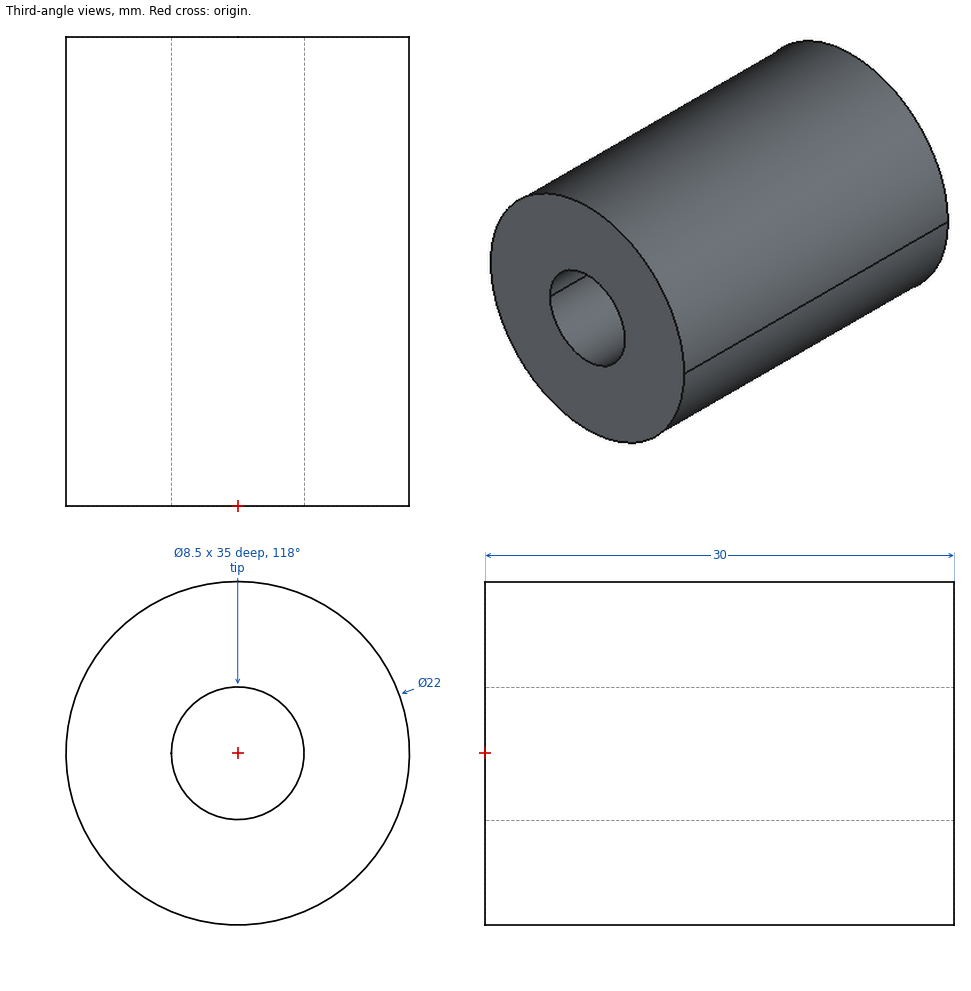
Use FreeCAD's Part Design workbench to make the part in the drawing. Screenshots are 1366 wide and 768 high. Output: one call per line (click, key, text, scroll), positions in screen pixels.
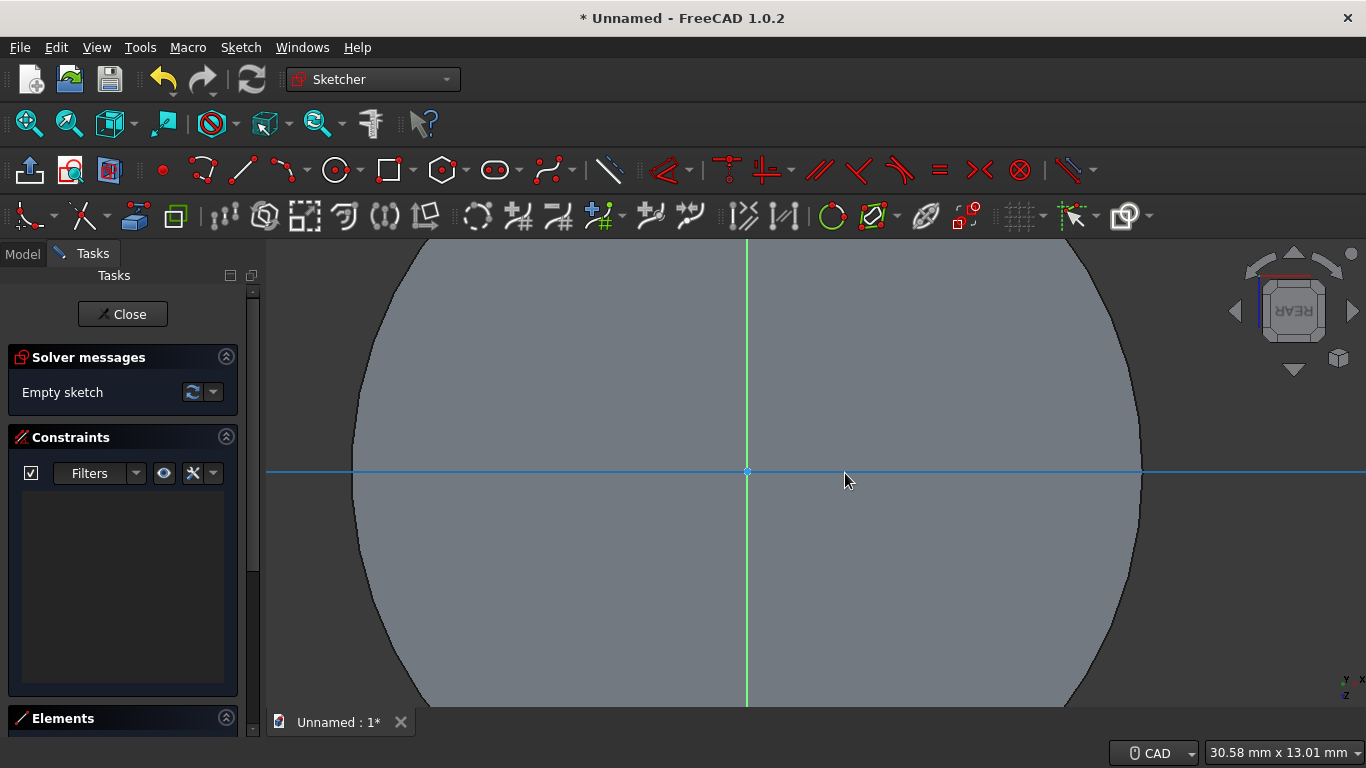
click(336, 170)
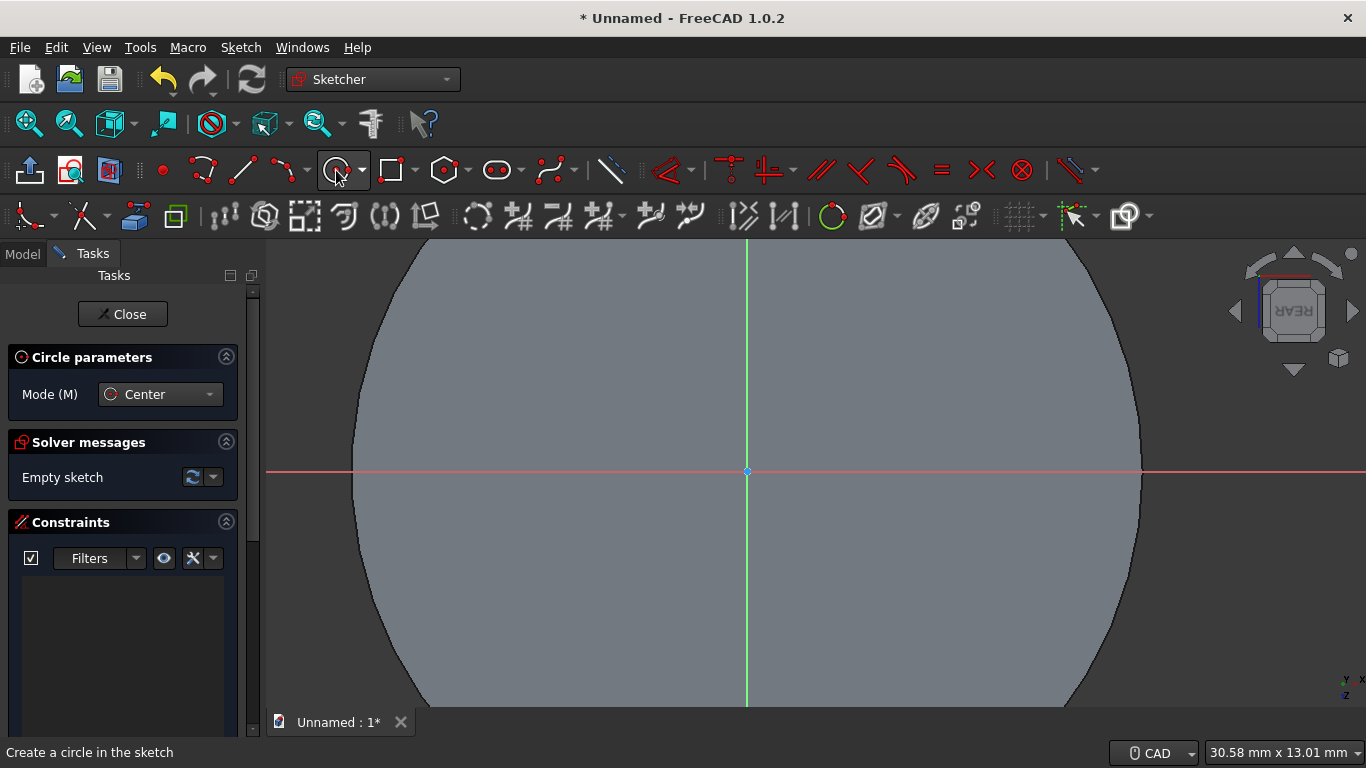
click(747, 472)
click(855, 364)
key(Escape)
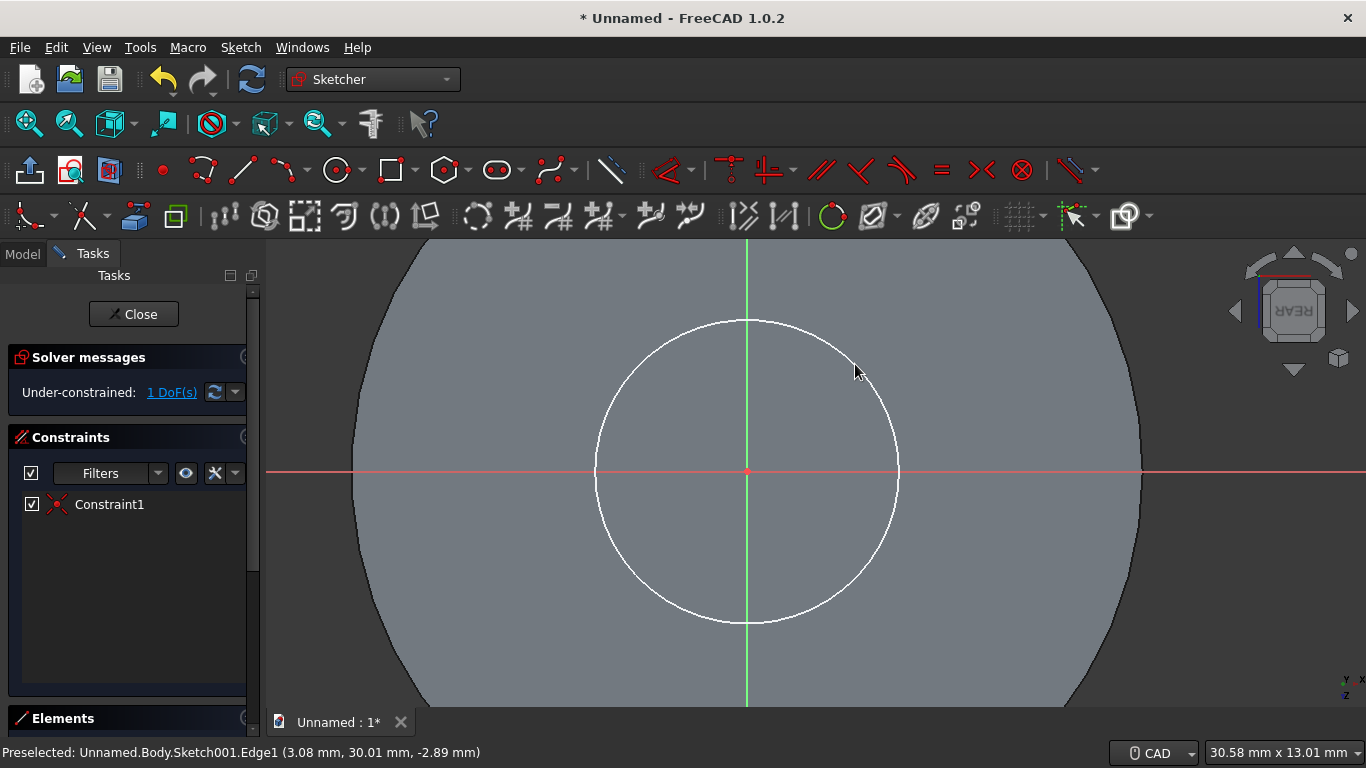
click(666, 170)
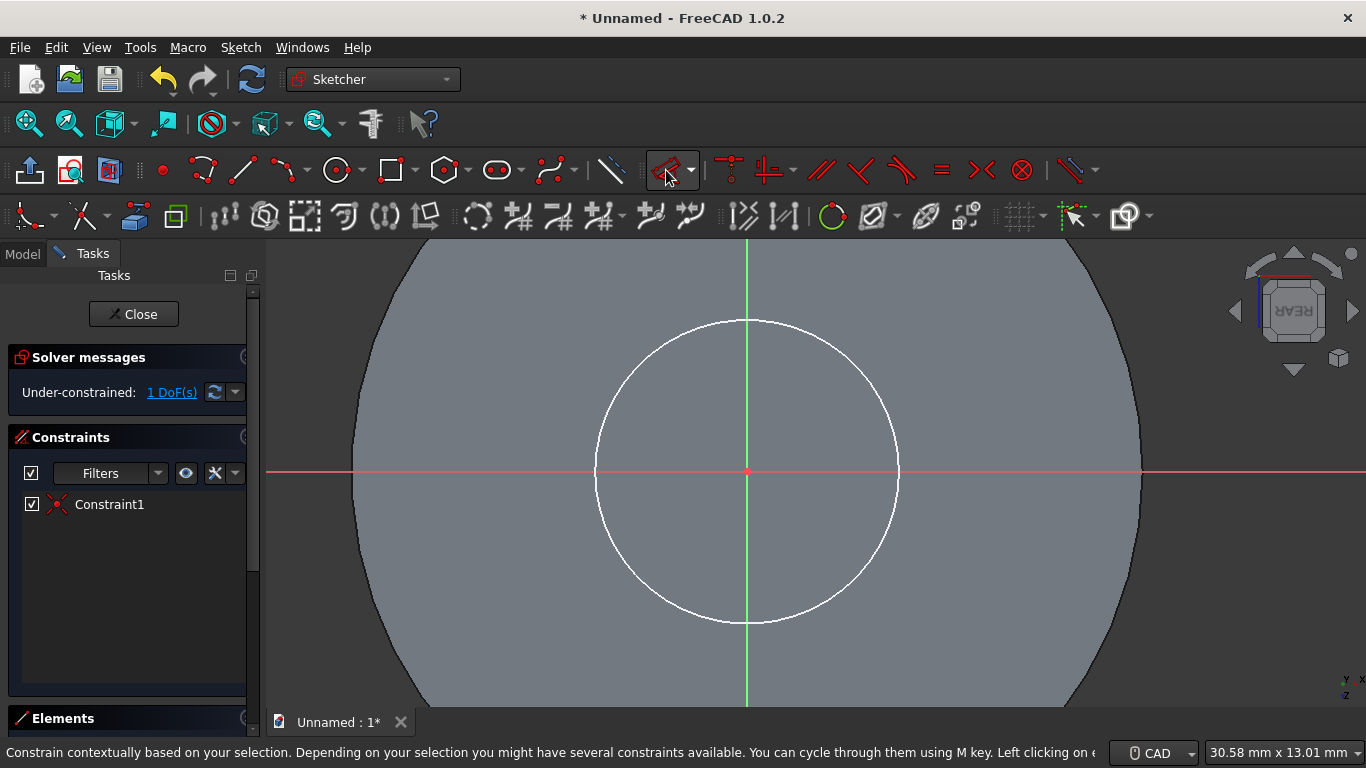
click(854, 364)
click(877, 341)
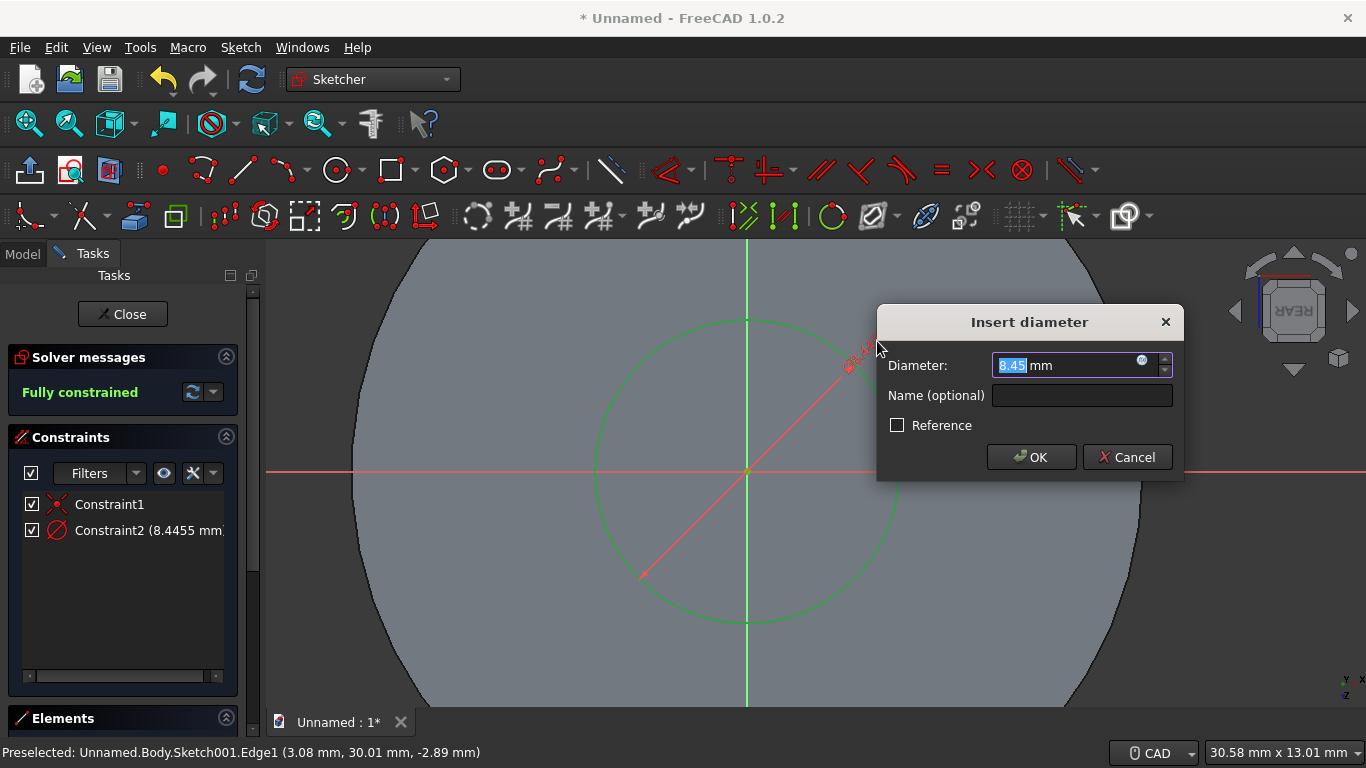
text(8.5)
key(Return)
key(Escape)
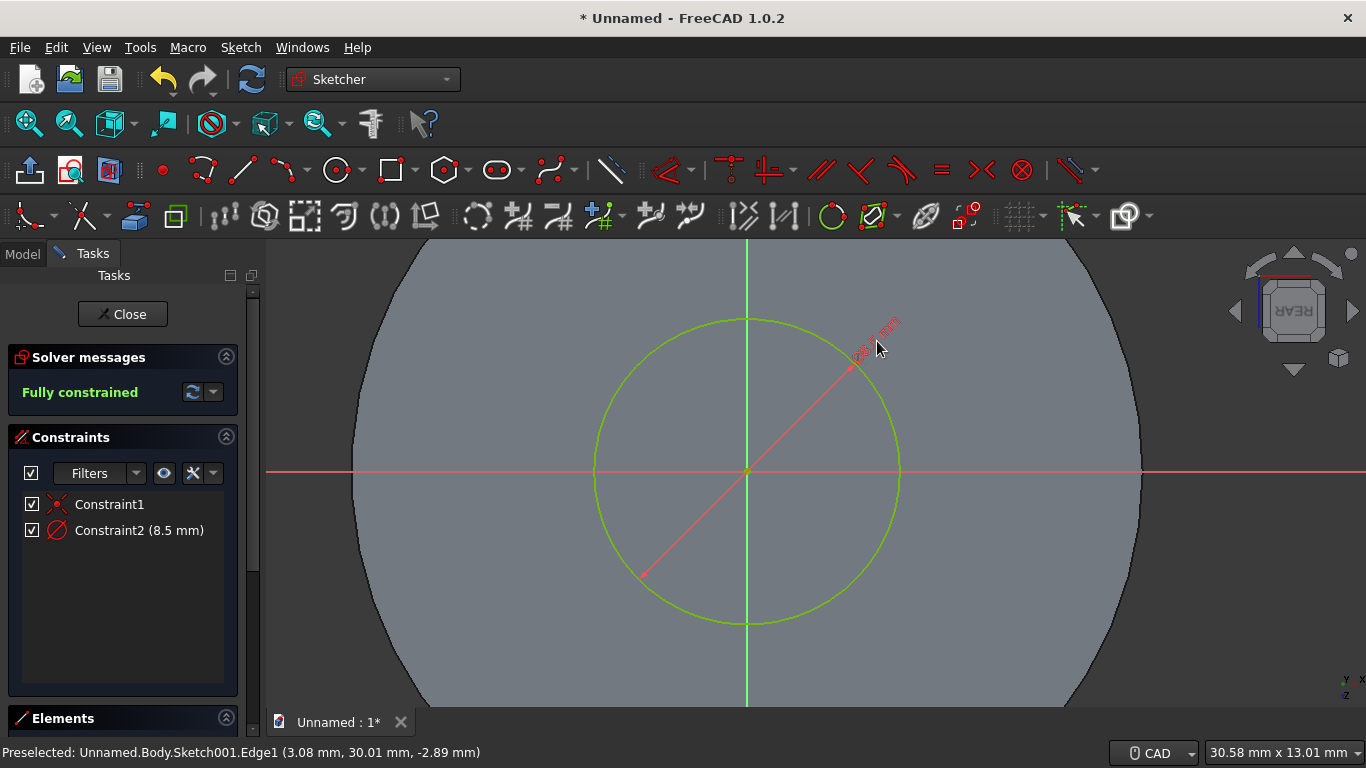
click(123, 314)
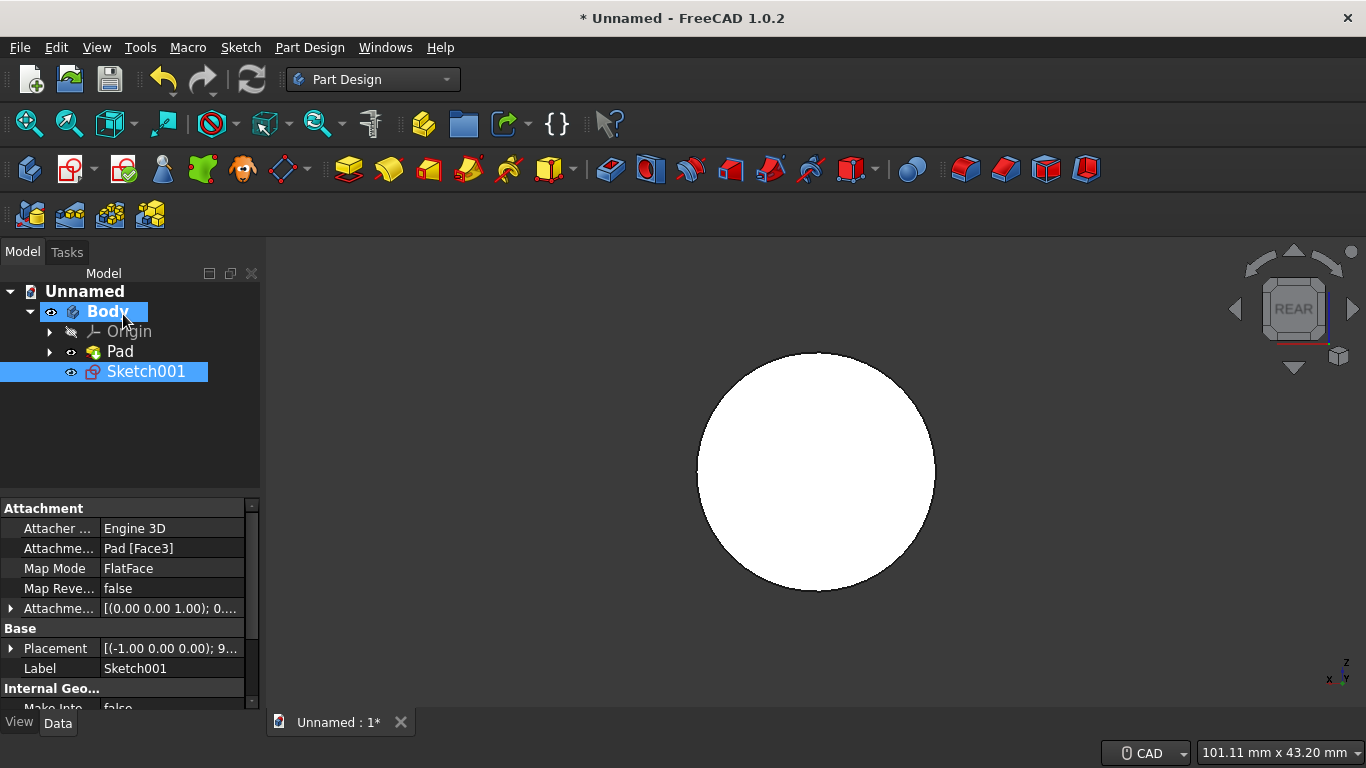
click(652, 170)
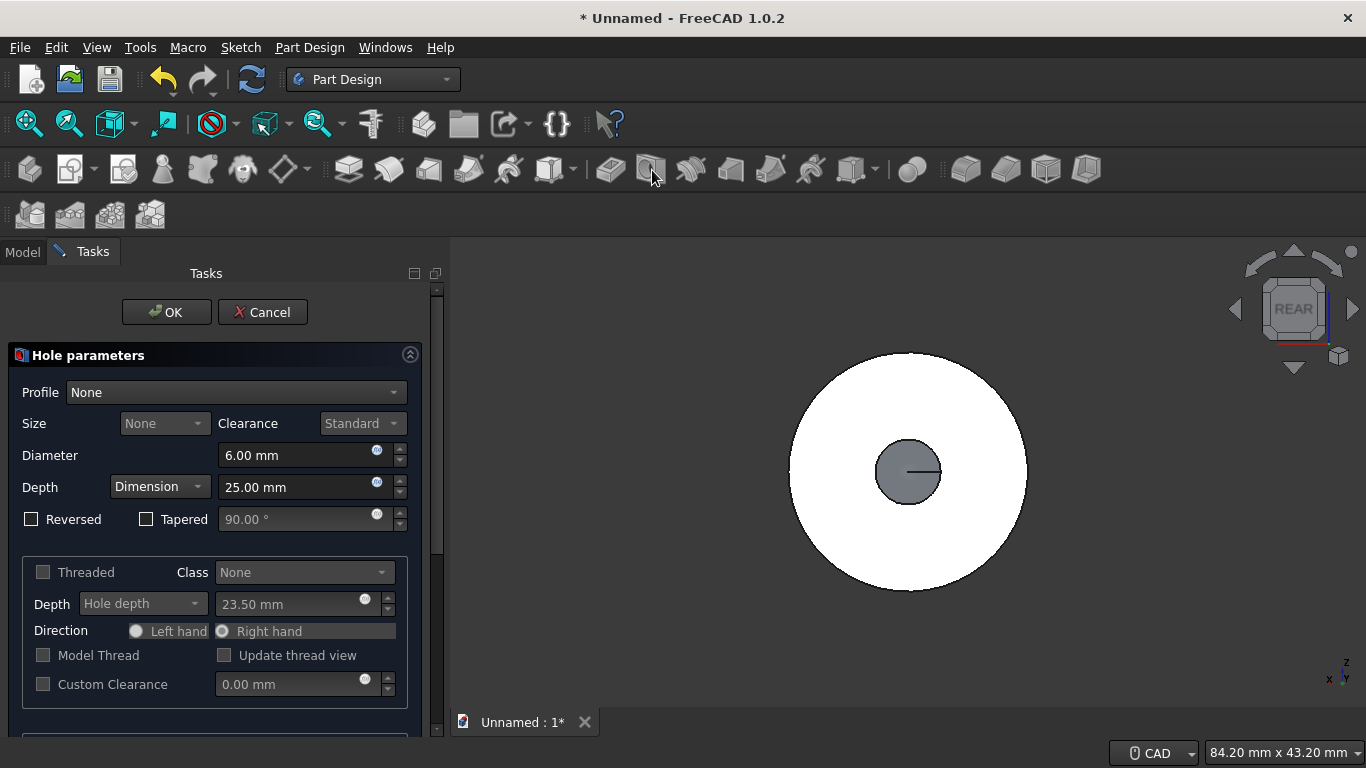
triple_click(305, 455)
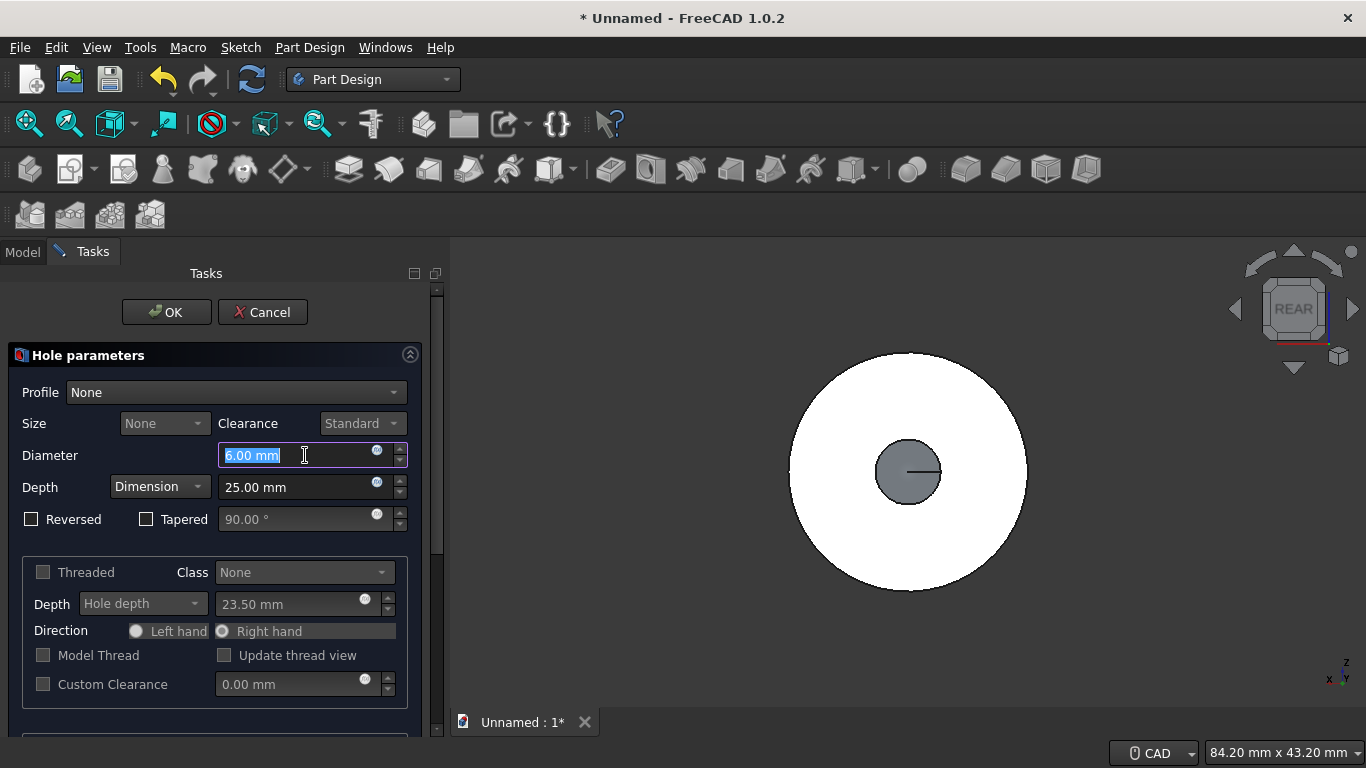
text(8.5)
key(Tab)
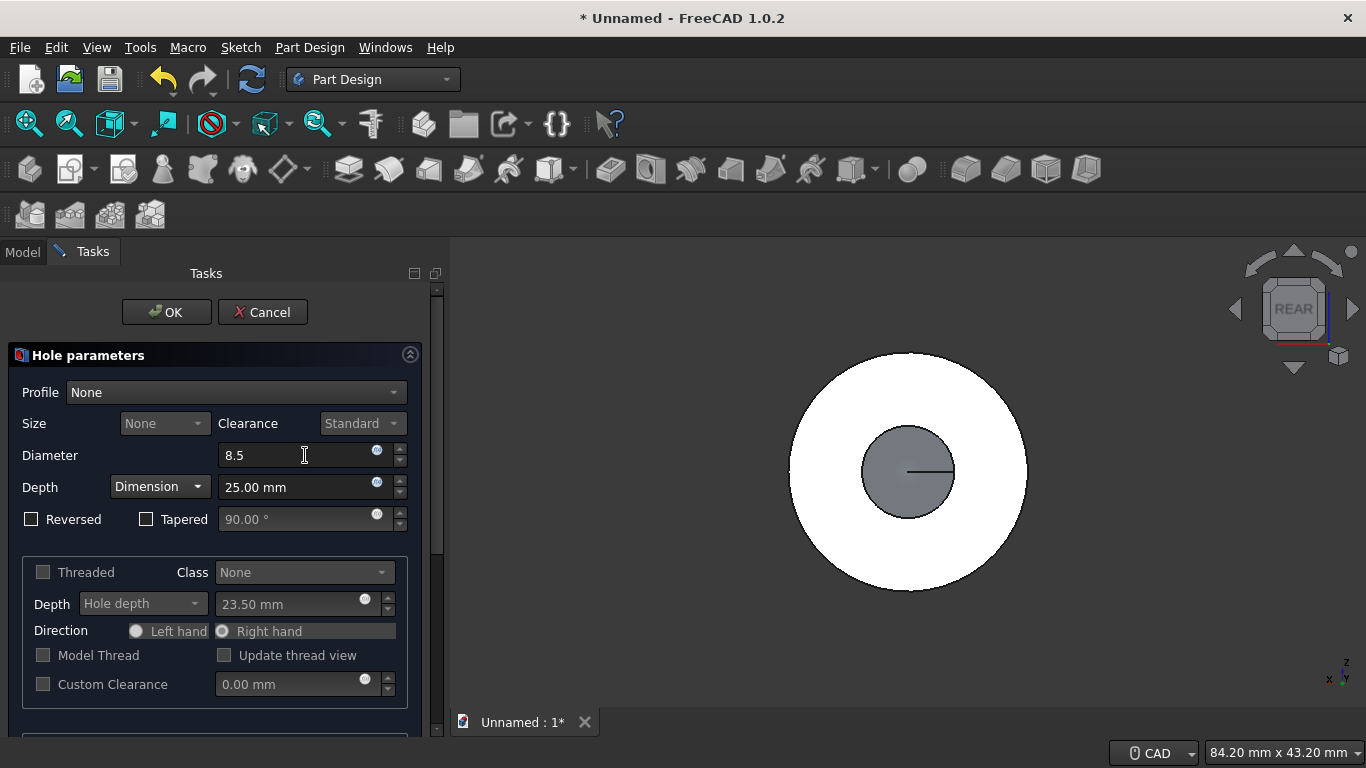
triple_click(305, 487)